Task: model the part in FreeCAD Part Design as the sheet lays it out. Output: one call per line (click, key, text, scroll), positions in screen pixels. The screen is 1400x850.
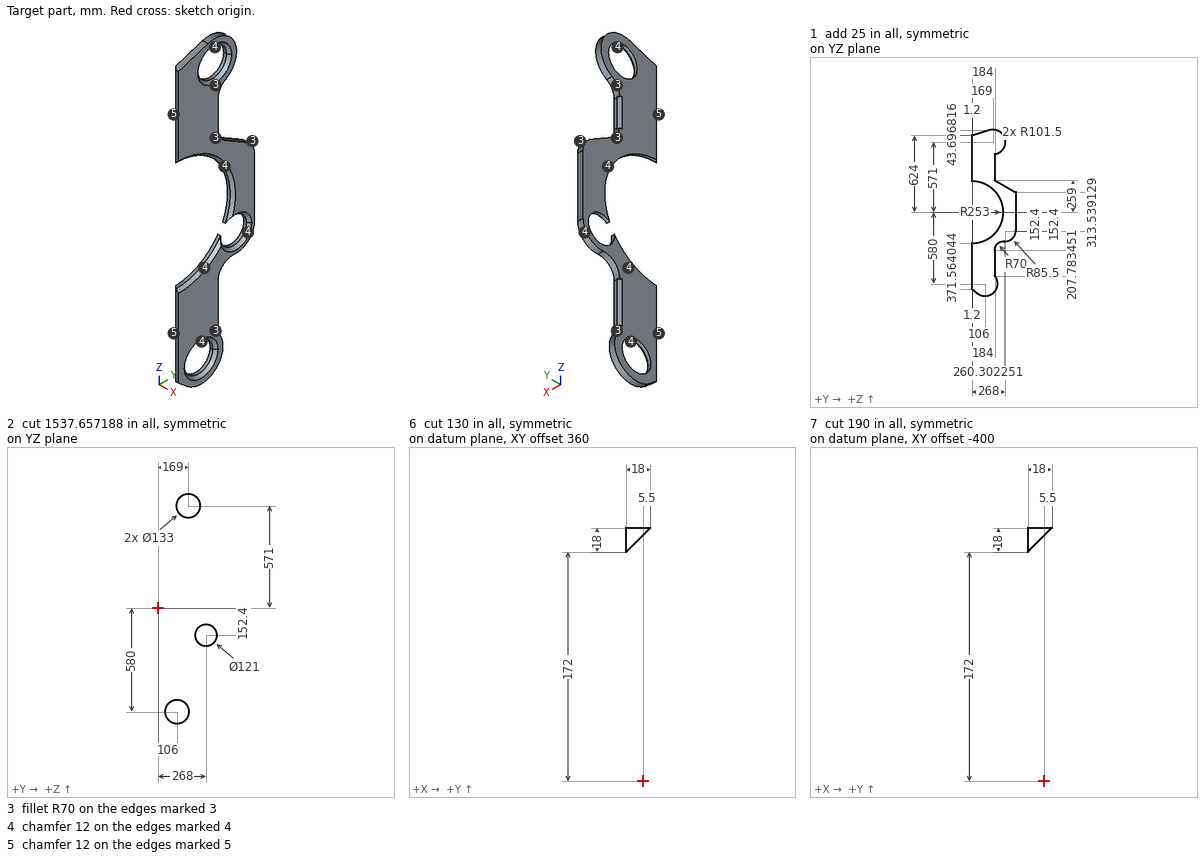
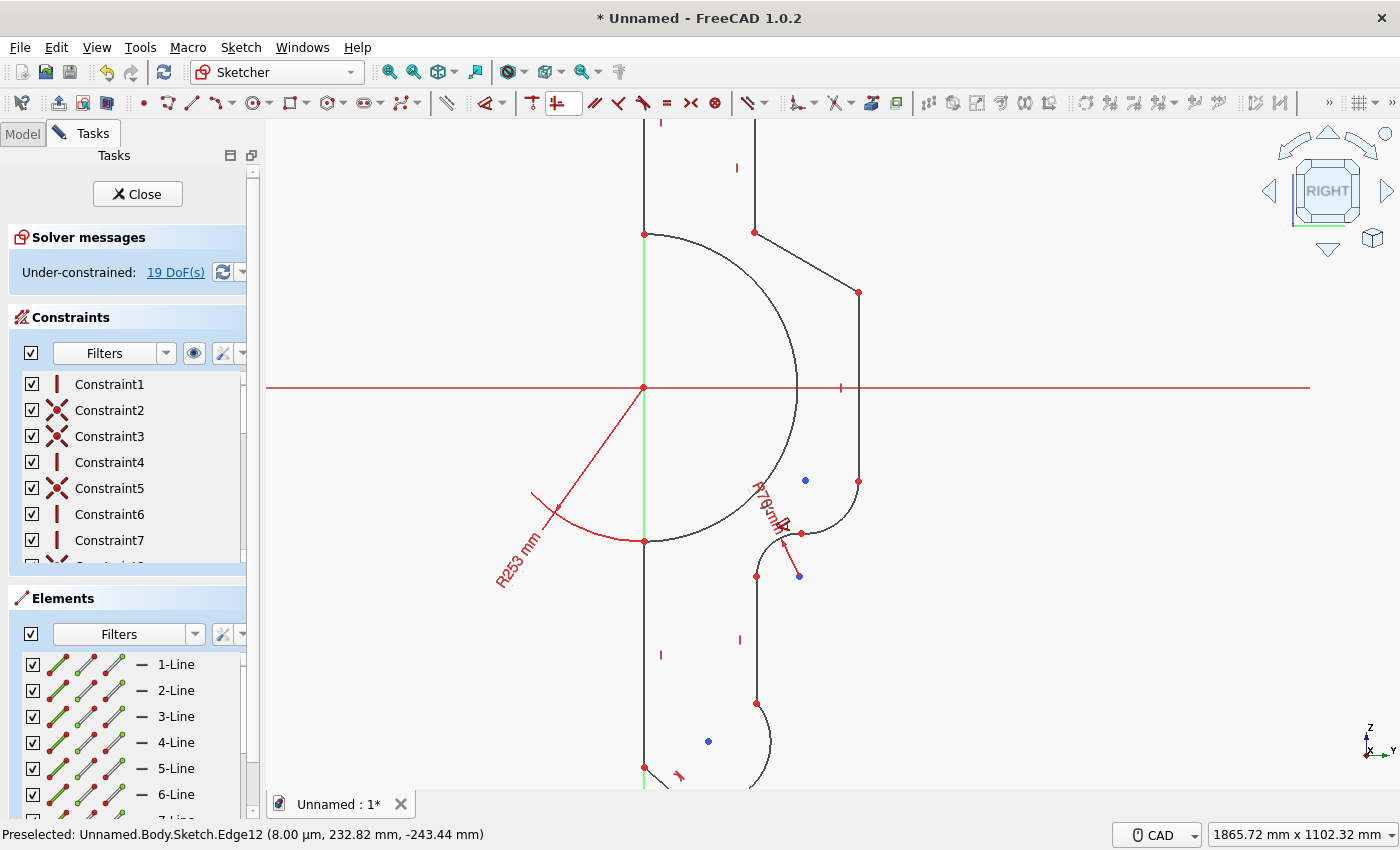
click(827, 529)
click(840, 558)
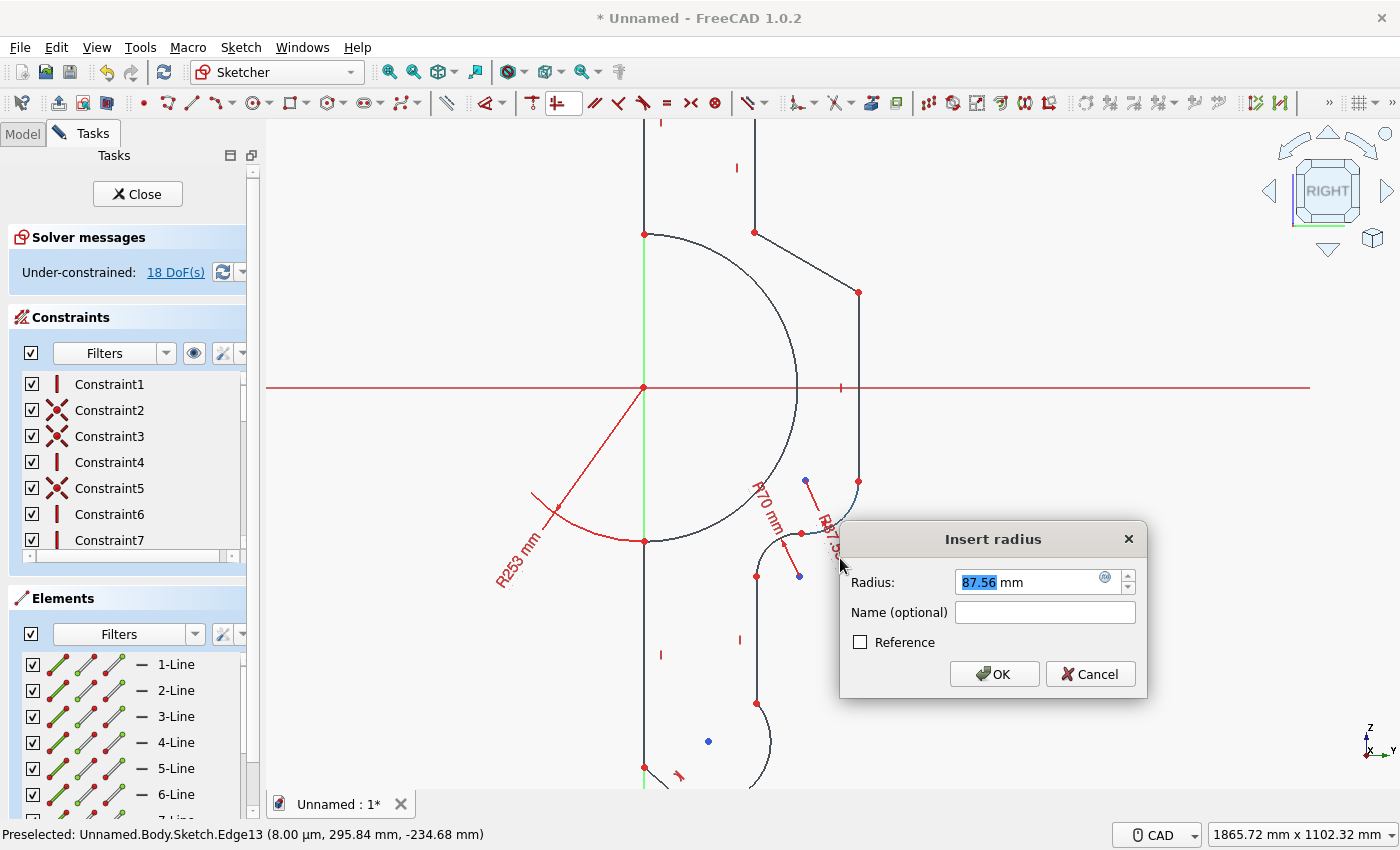
text(85.5)
key(Return)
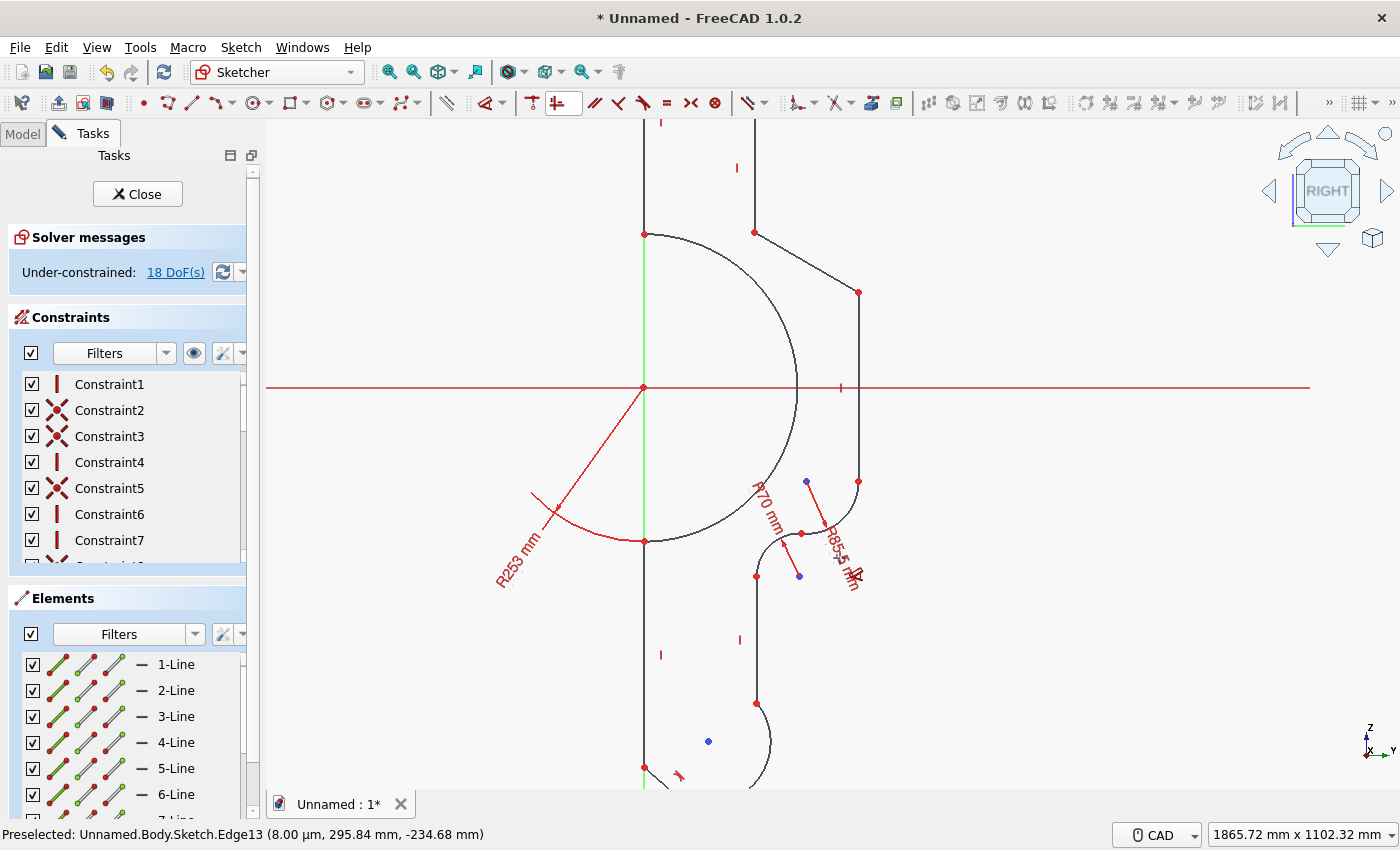
click(755, 232)
click(699, 198)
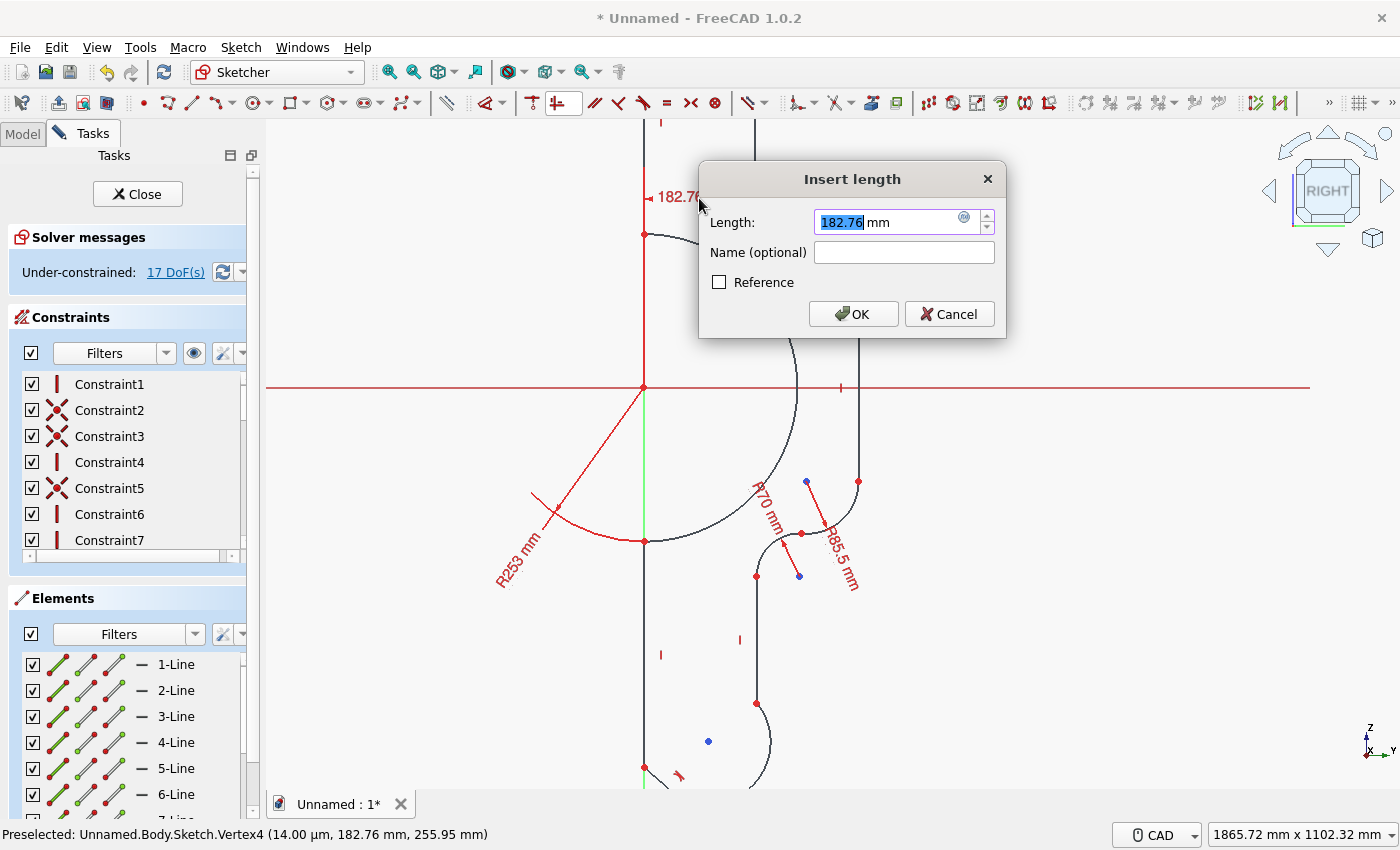
text(184)
key(Return)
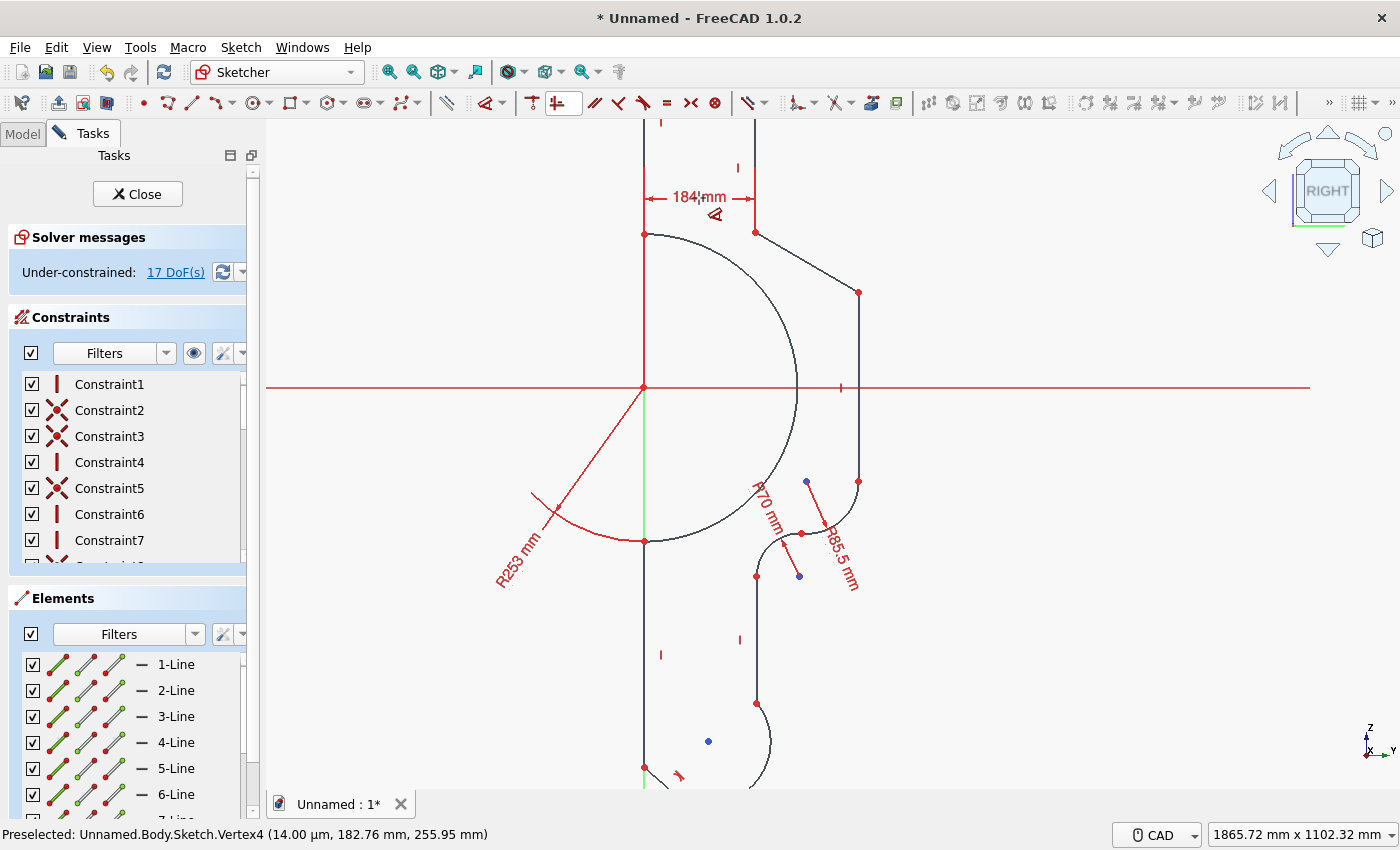
click(755, 232)
click(610, 310)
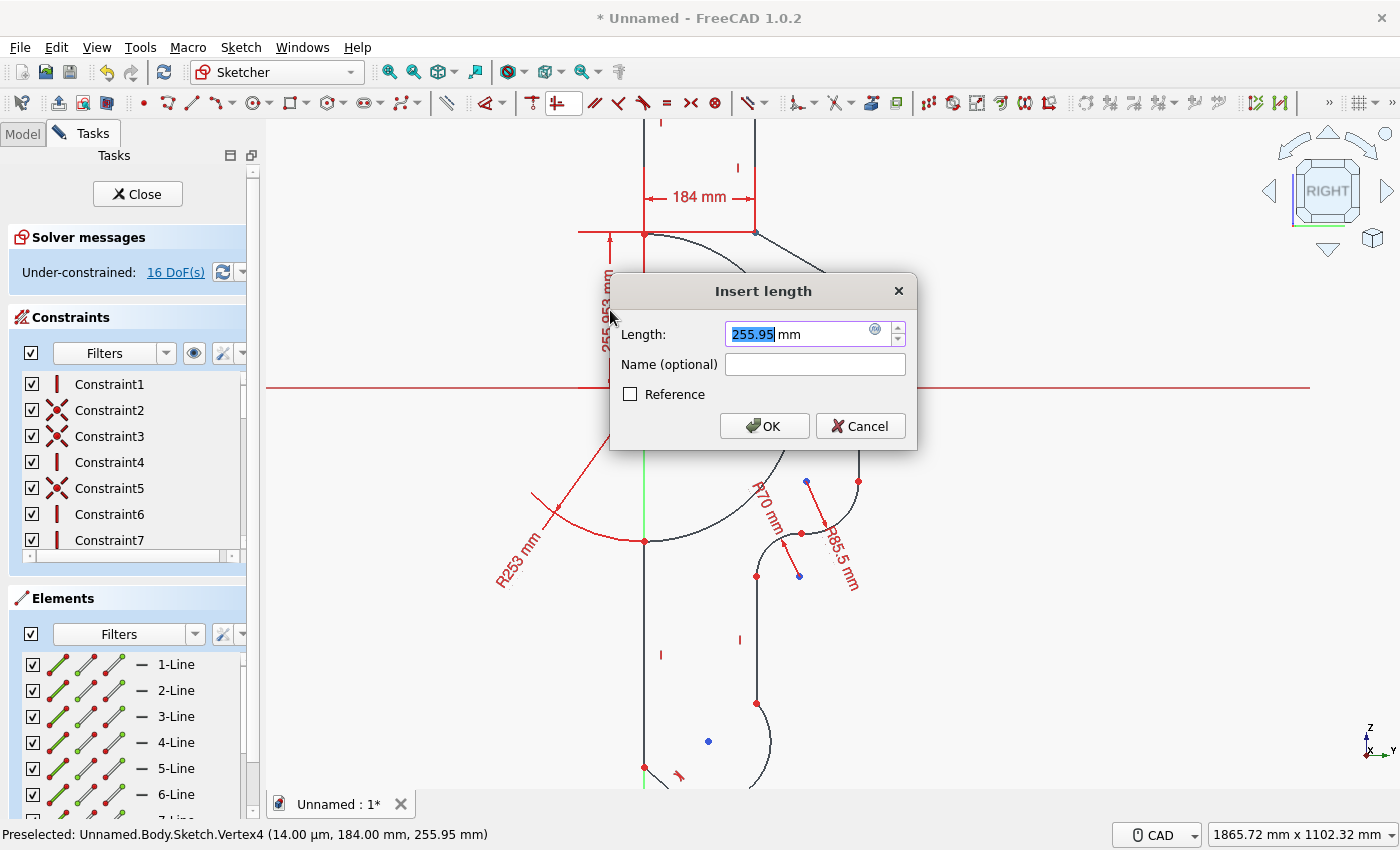
text(259)
key(Return)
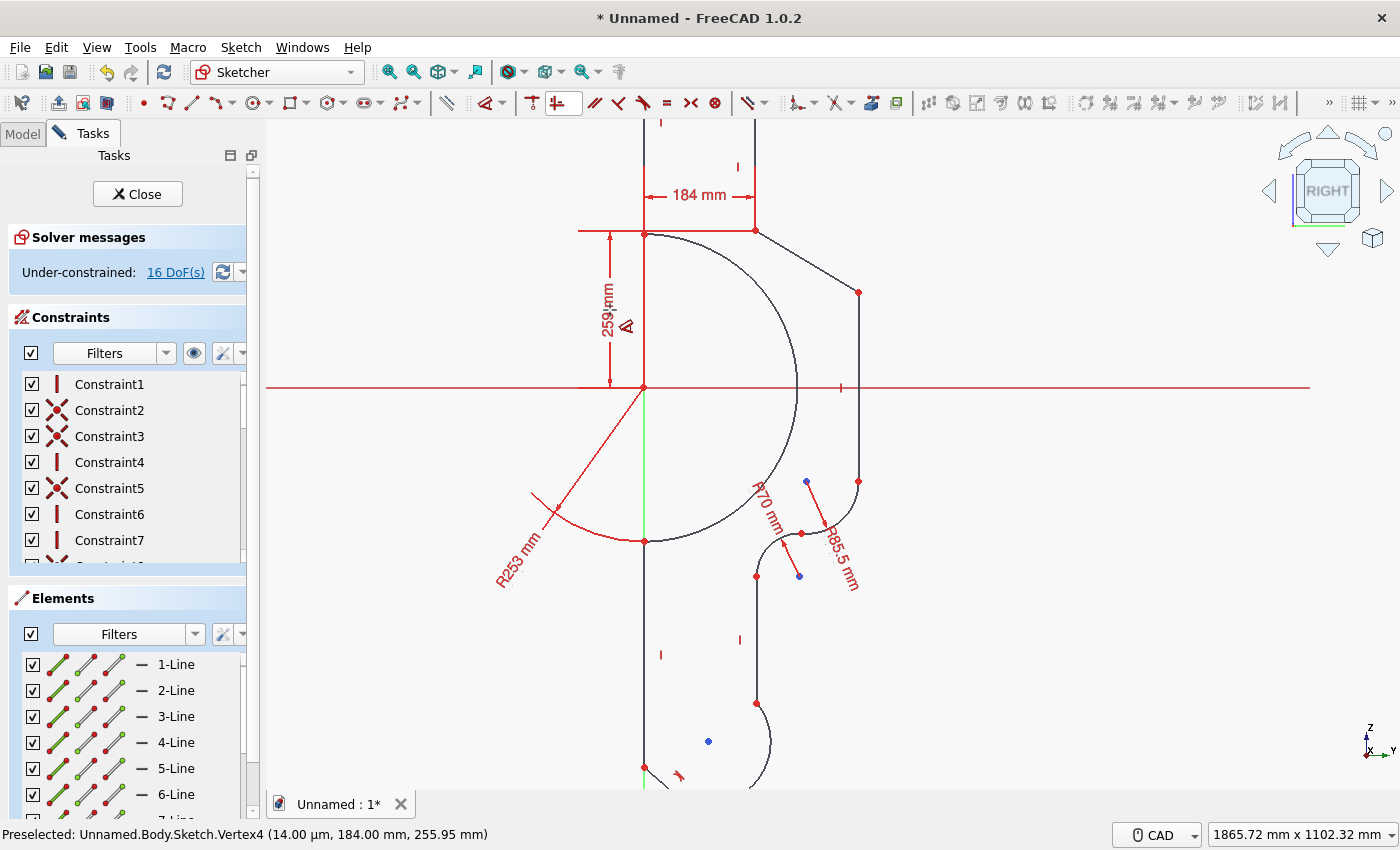
scroll(781, 538, down, 3)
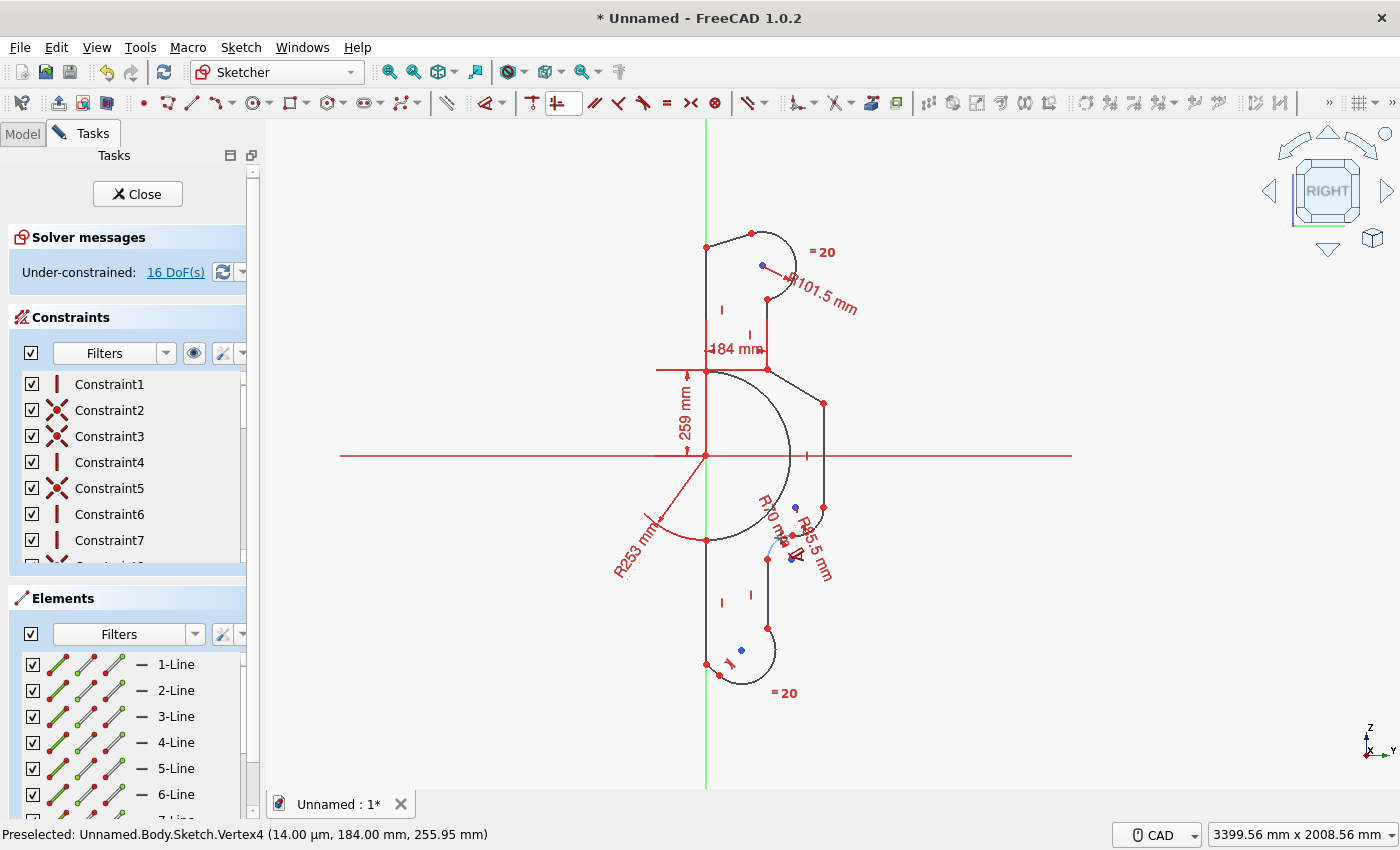
scroll(706, 248, up, 23)